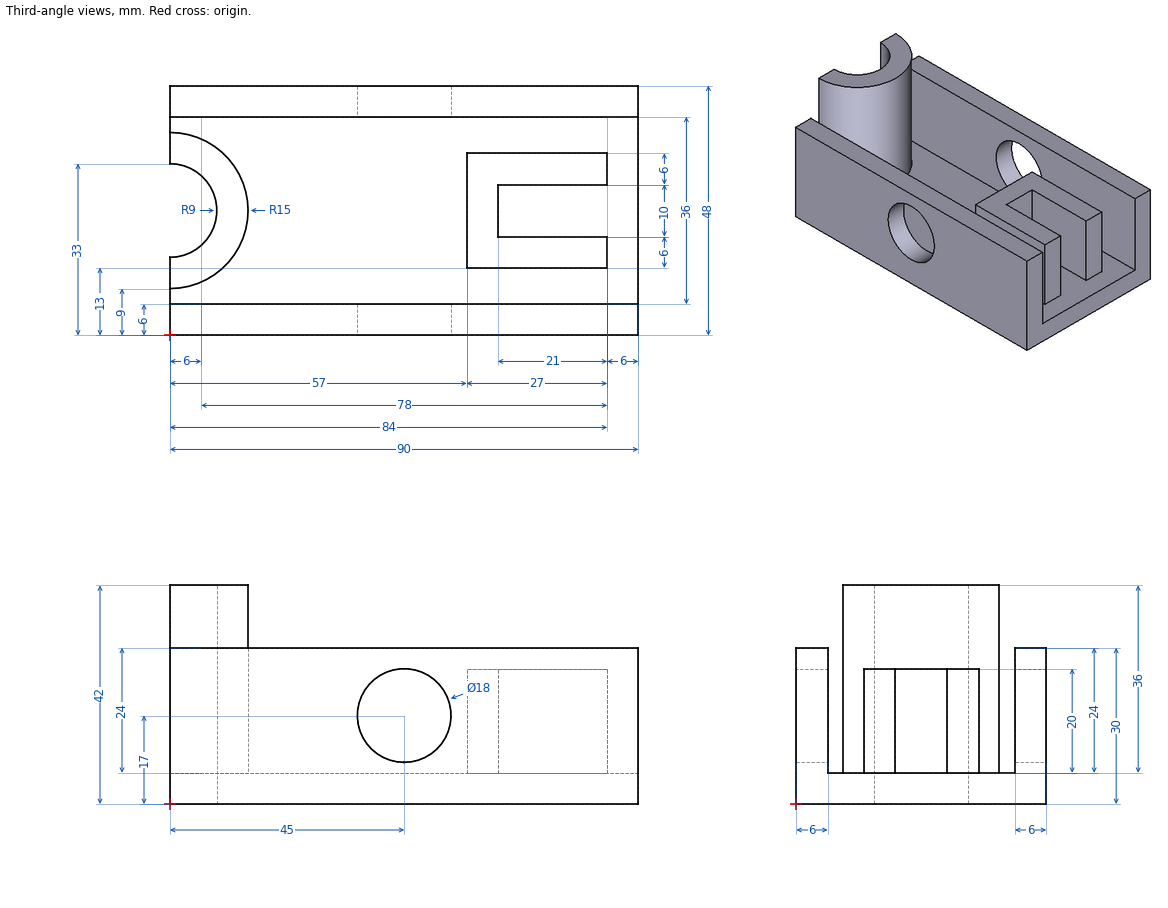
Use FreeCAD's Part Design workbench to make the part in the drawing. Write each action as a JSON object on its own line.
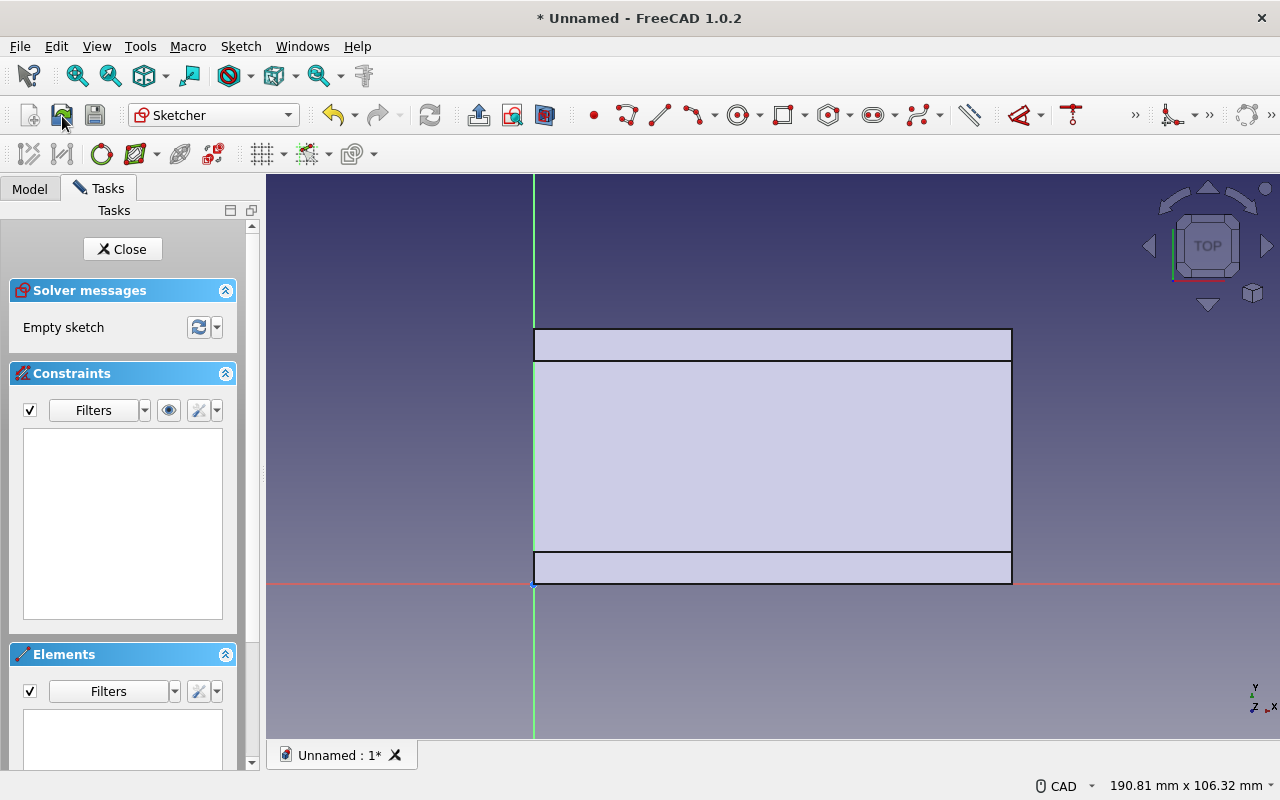
{"action": "scroll", "coordinate": [415, 510], "scroll_direction": "up", "scroll_amount": 3}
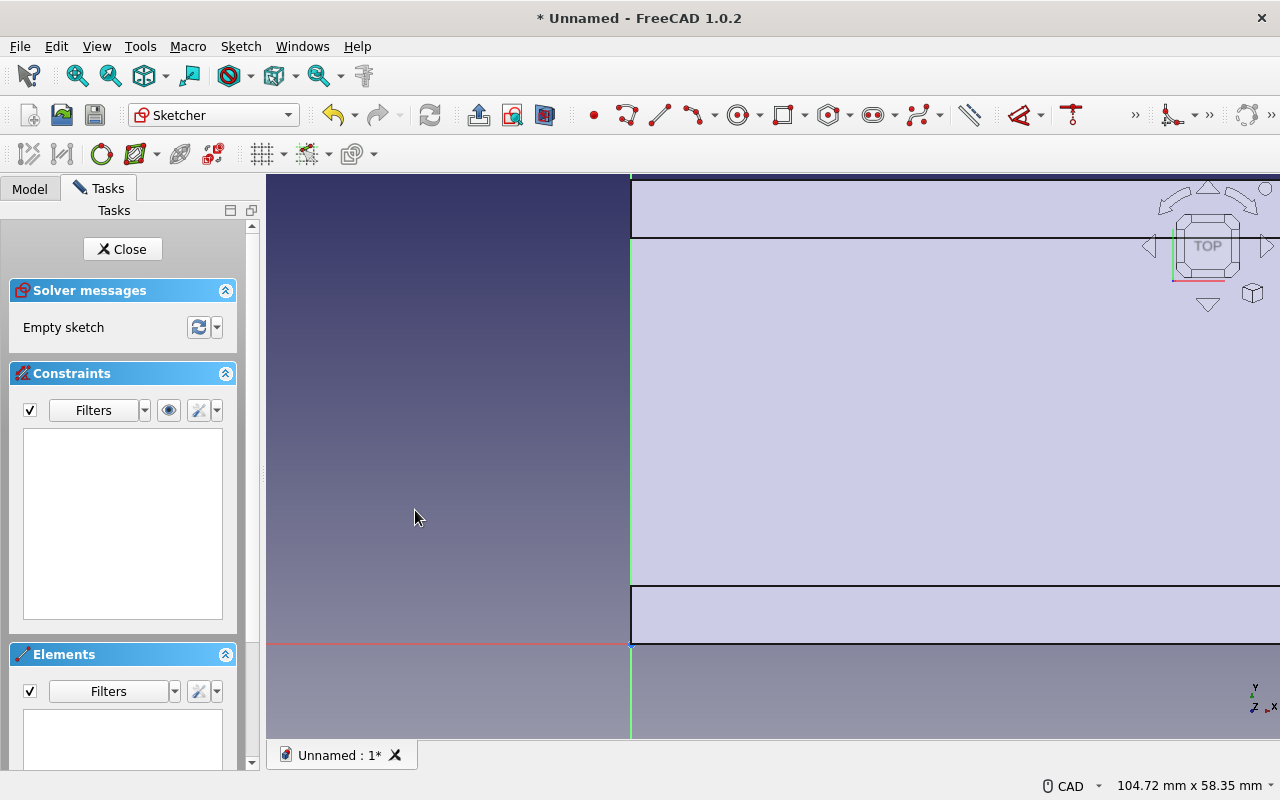
{"action": "key", "text": "g l"}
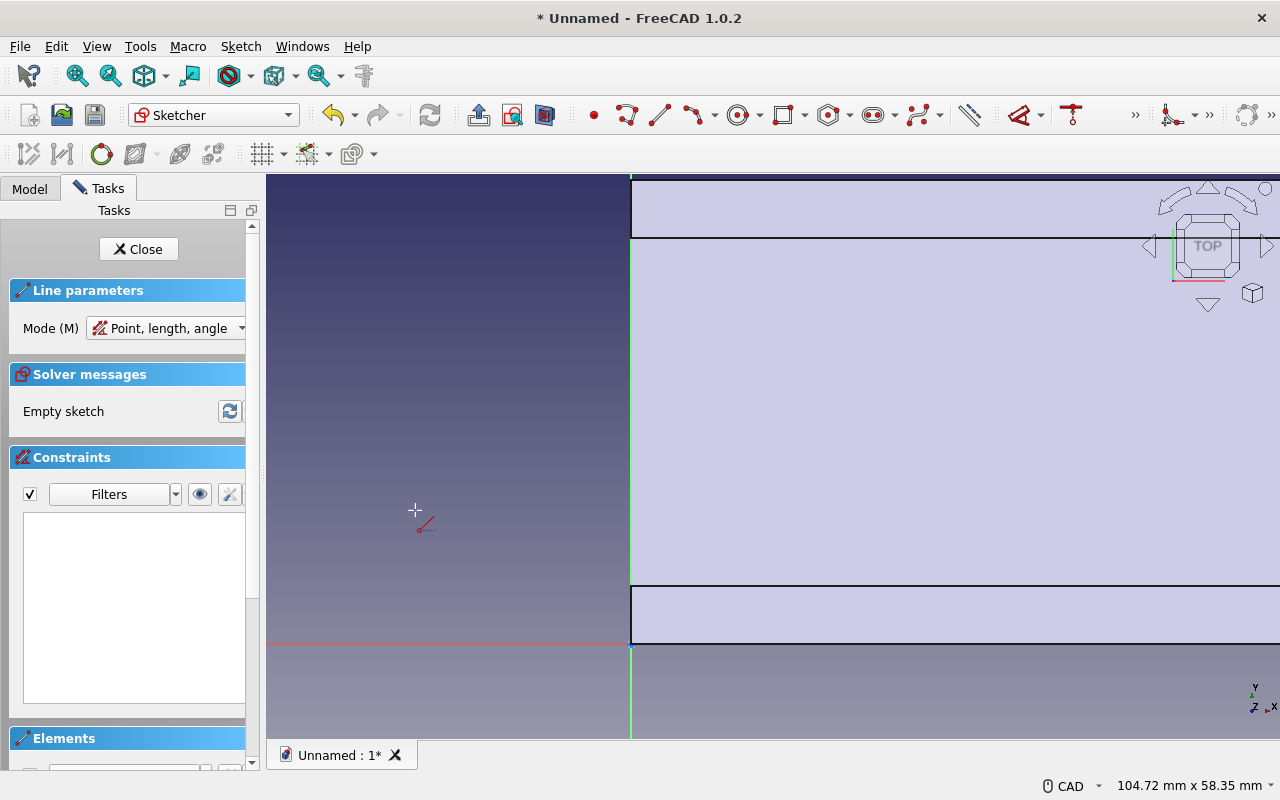
{"action": "left_click", "coordinate": [631, 267]}
{"action": "left_click", "coordinate": [640, 557]}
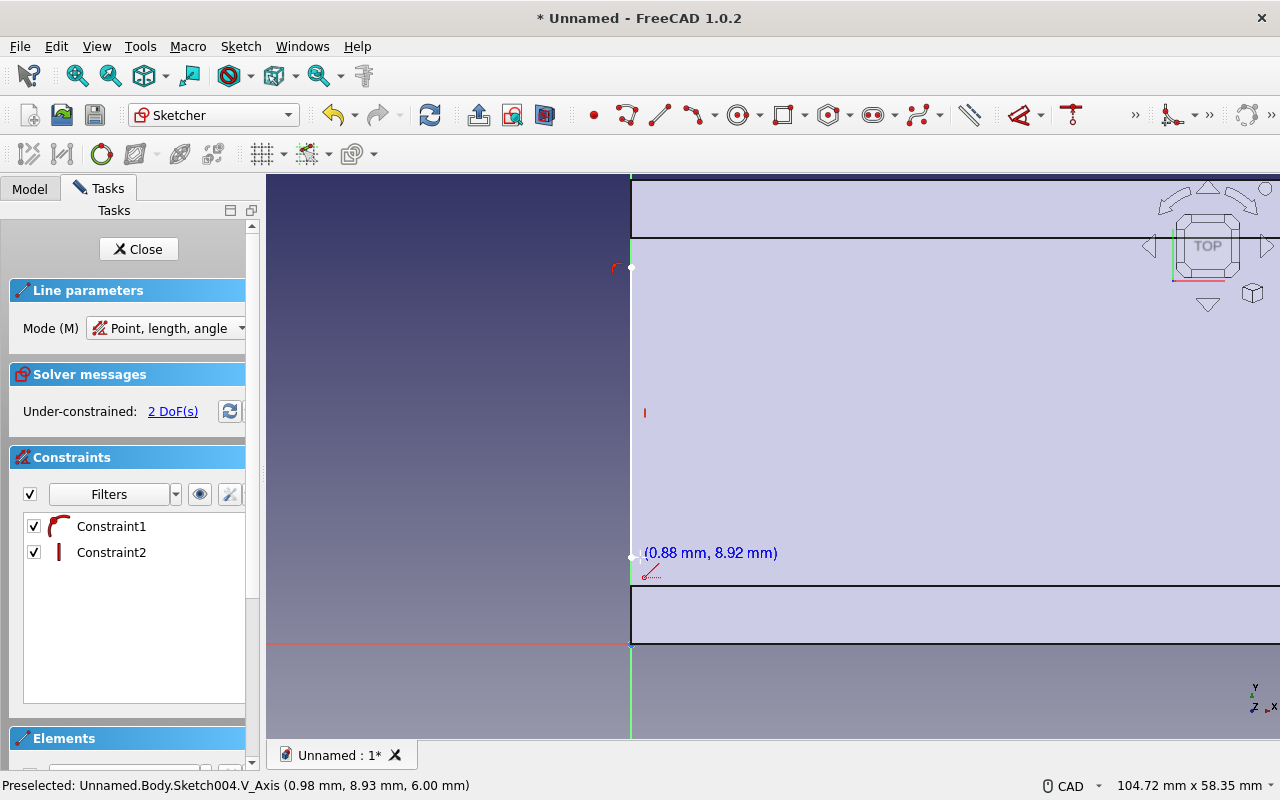
{"action": "key", "text": "g 3 a"}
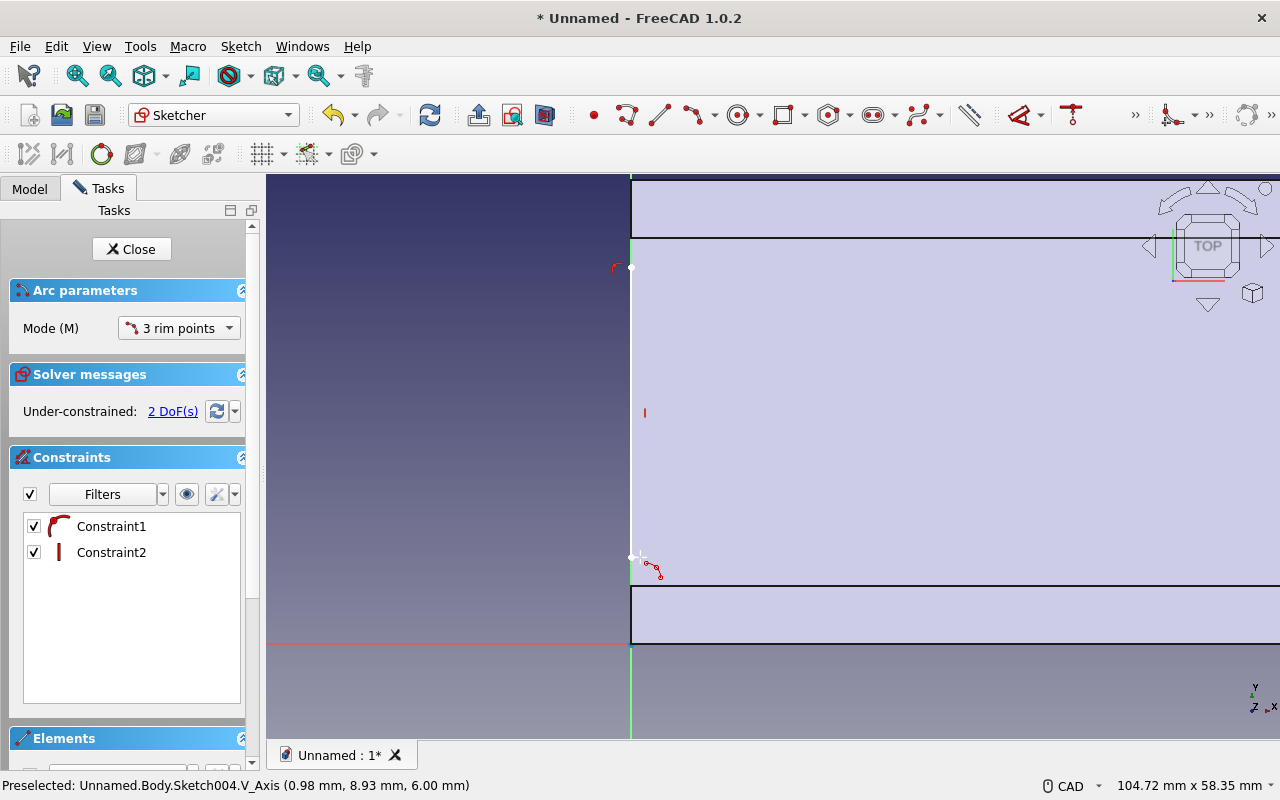
{"action": "left_click", "coordinate": [631, 558]}
{"action": "left_click", "coordinate": [631, 268]}
{"action": "left_click", "coordinate": [777, 412]}
{"action": "key", "text": "Escape"}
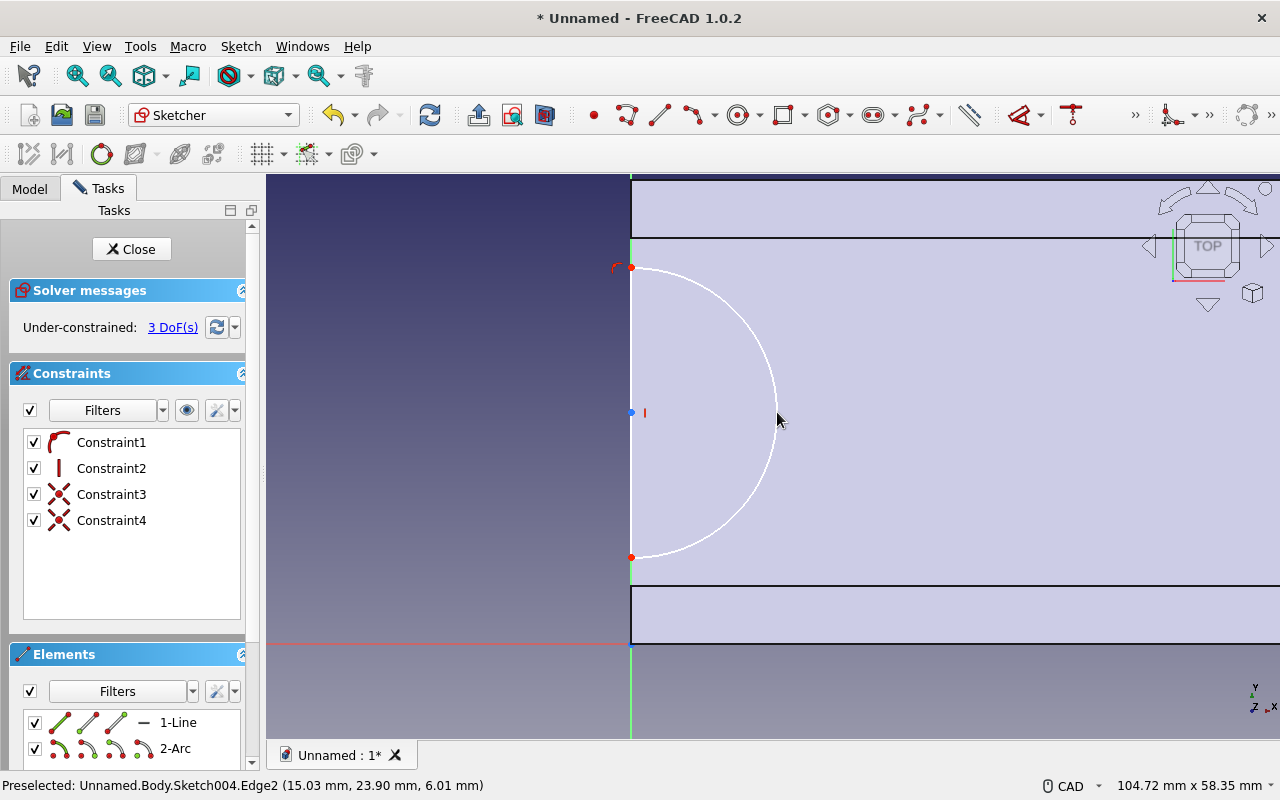
{"action": "left_click", "coordinate": [632, 413]}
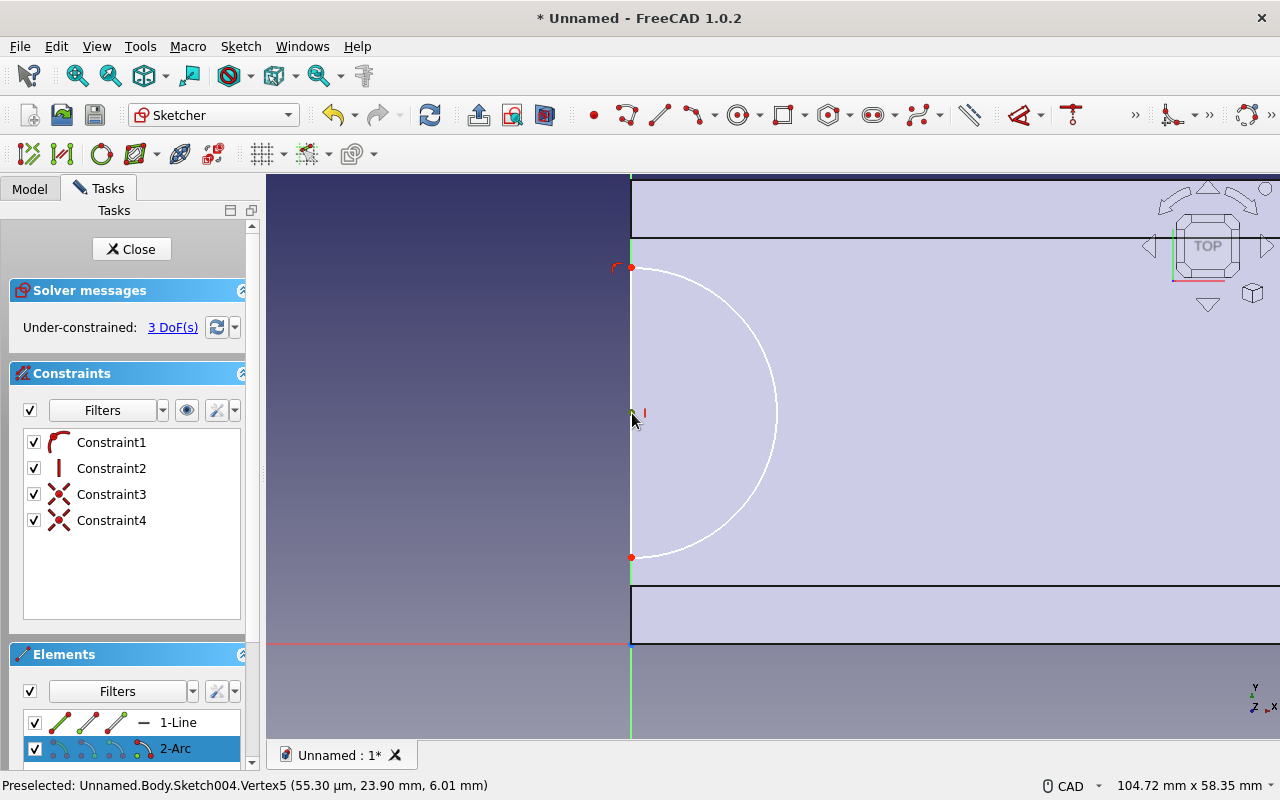
{"action": "left_click", "coordinate": [631, 675]}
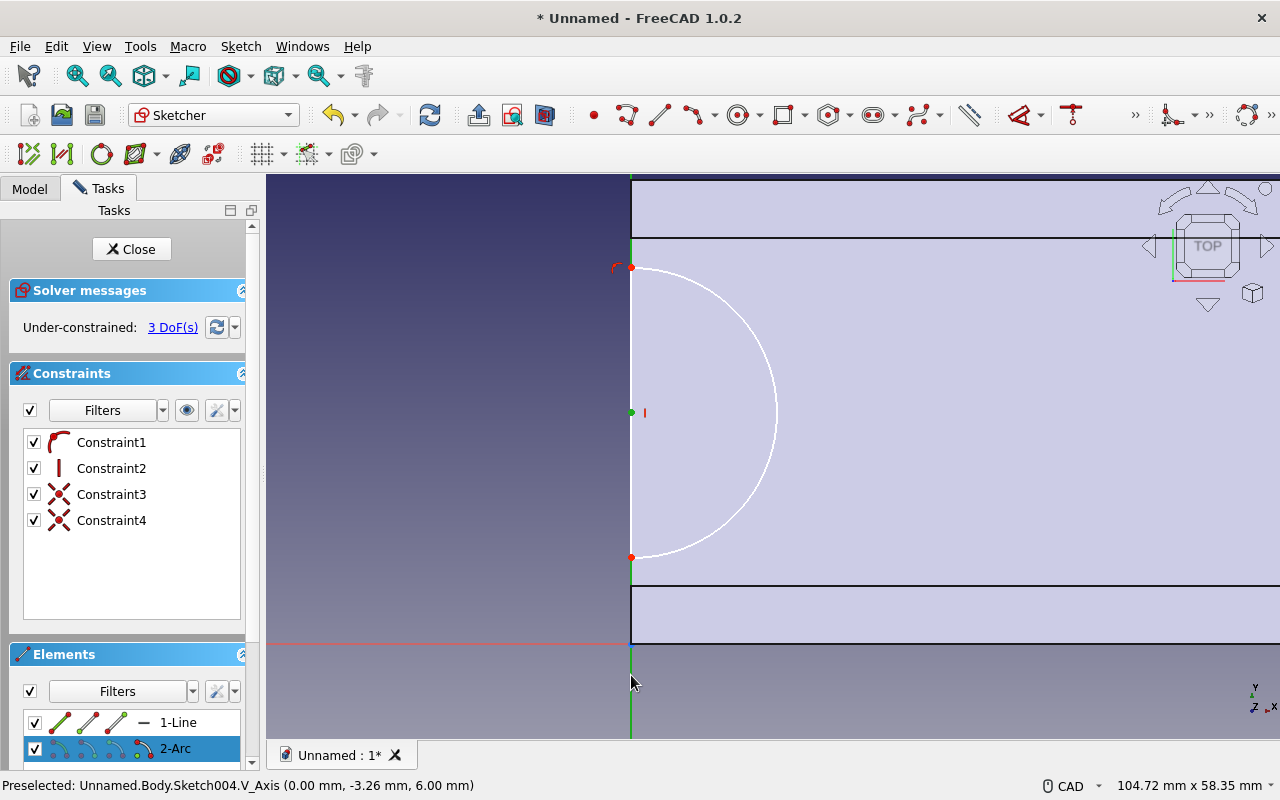
{"action": "key", "text": "c"}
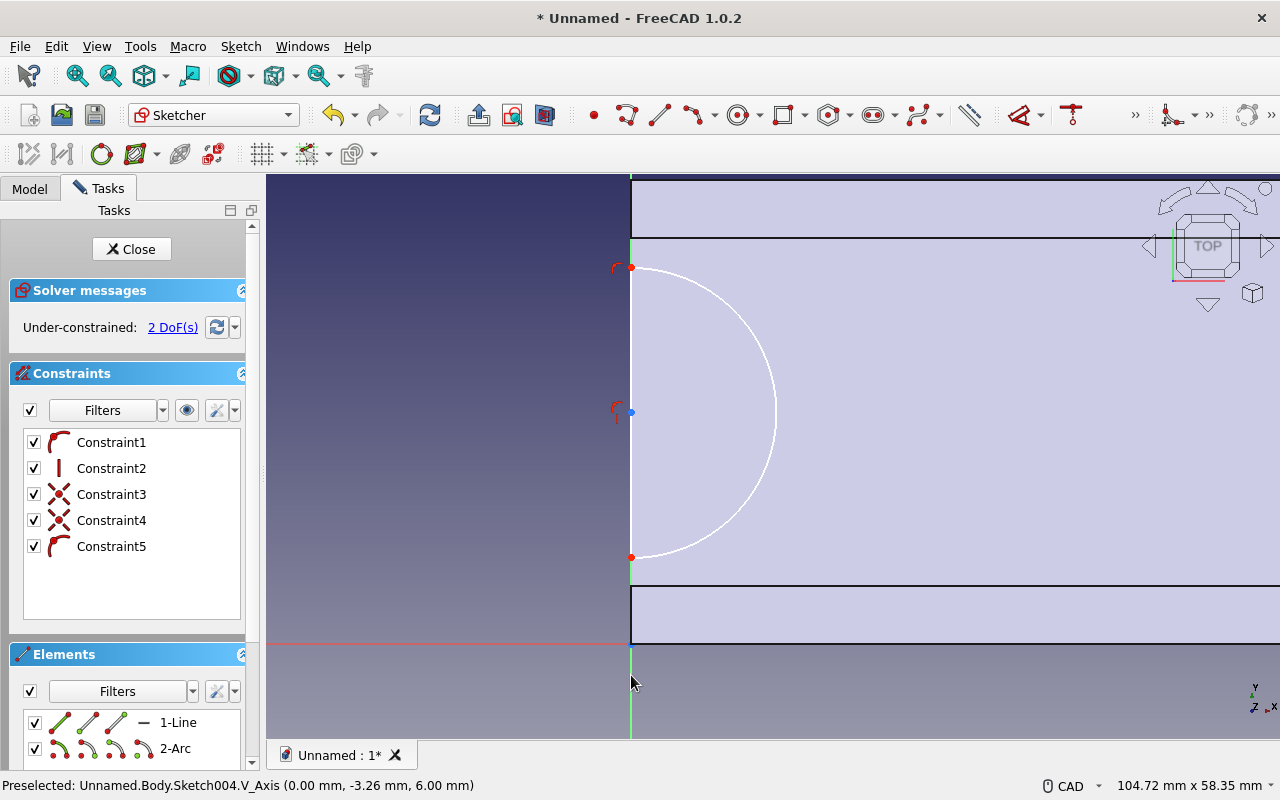
{"action": "key", "text": "d"}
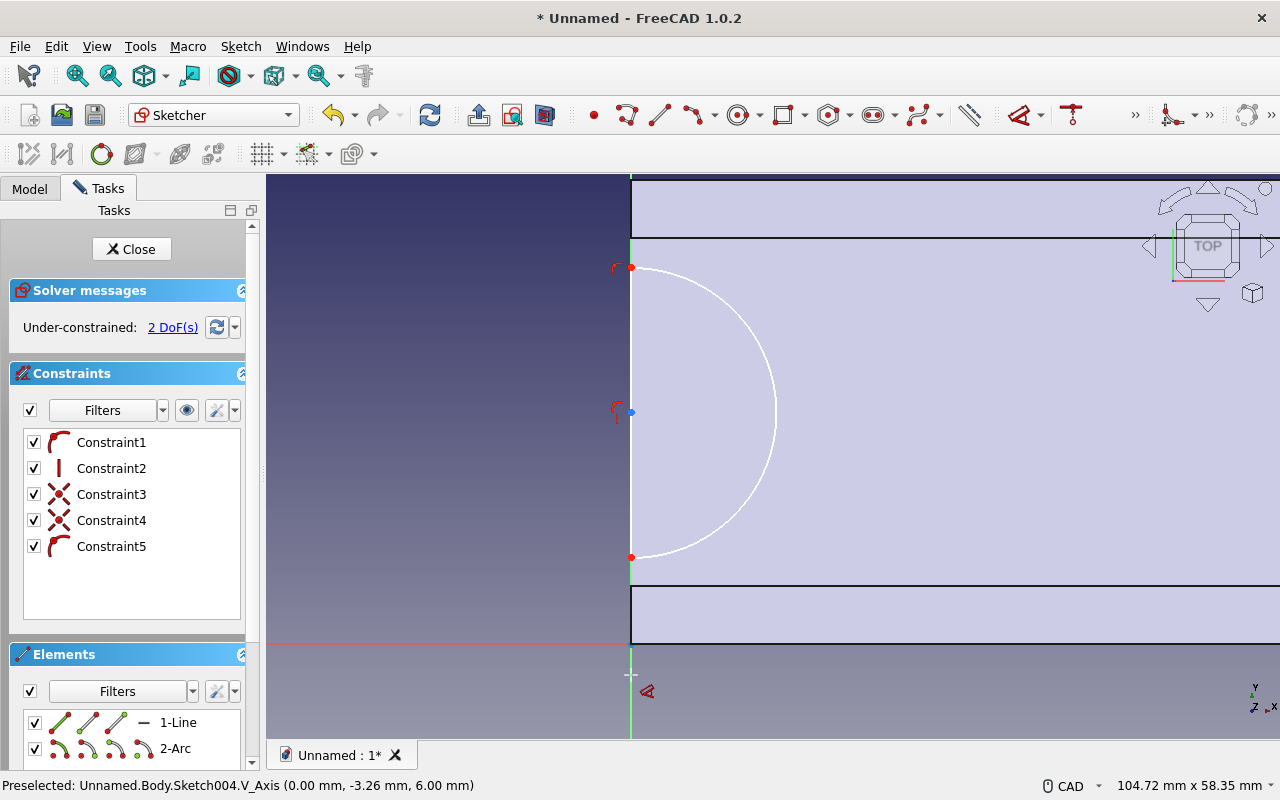
{"action": "left_click", "coordinate": [749, 498]}
{"action": "left_click", "coordinate": [775, 517]}